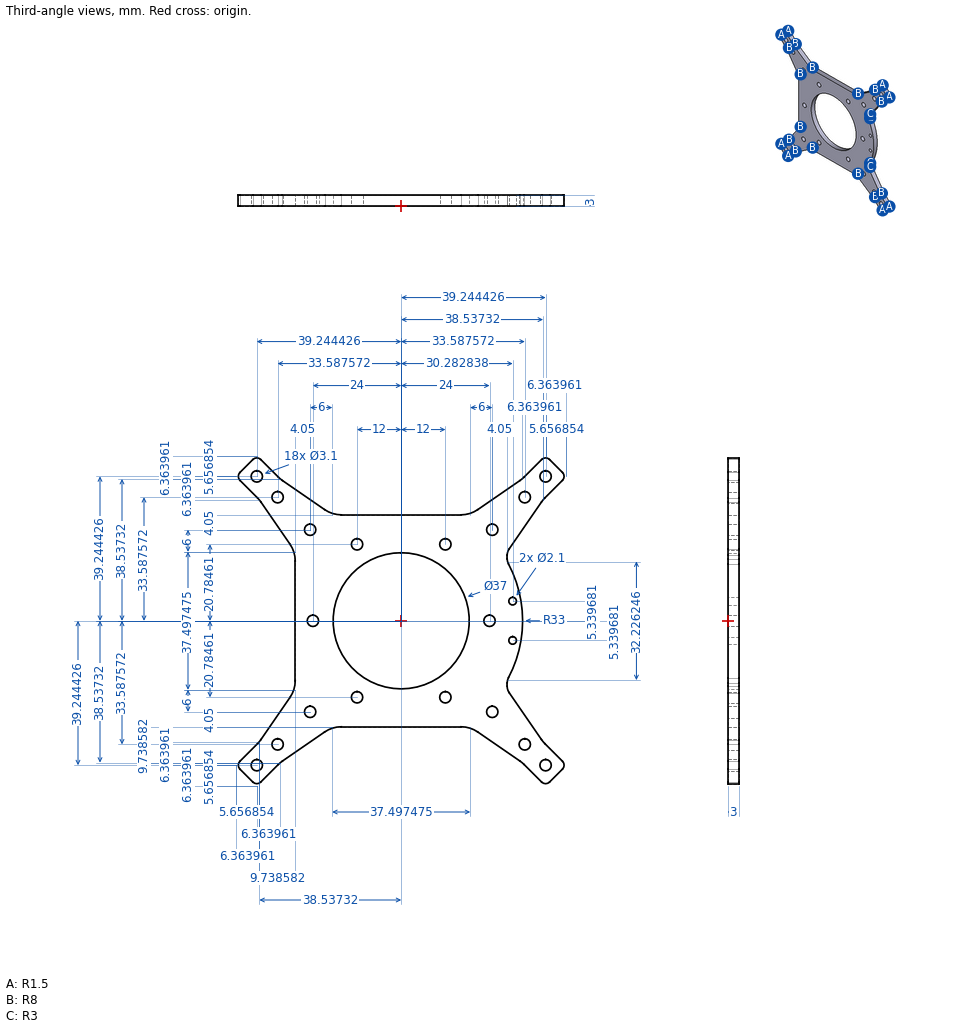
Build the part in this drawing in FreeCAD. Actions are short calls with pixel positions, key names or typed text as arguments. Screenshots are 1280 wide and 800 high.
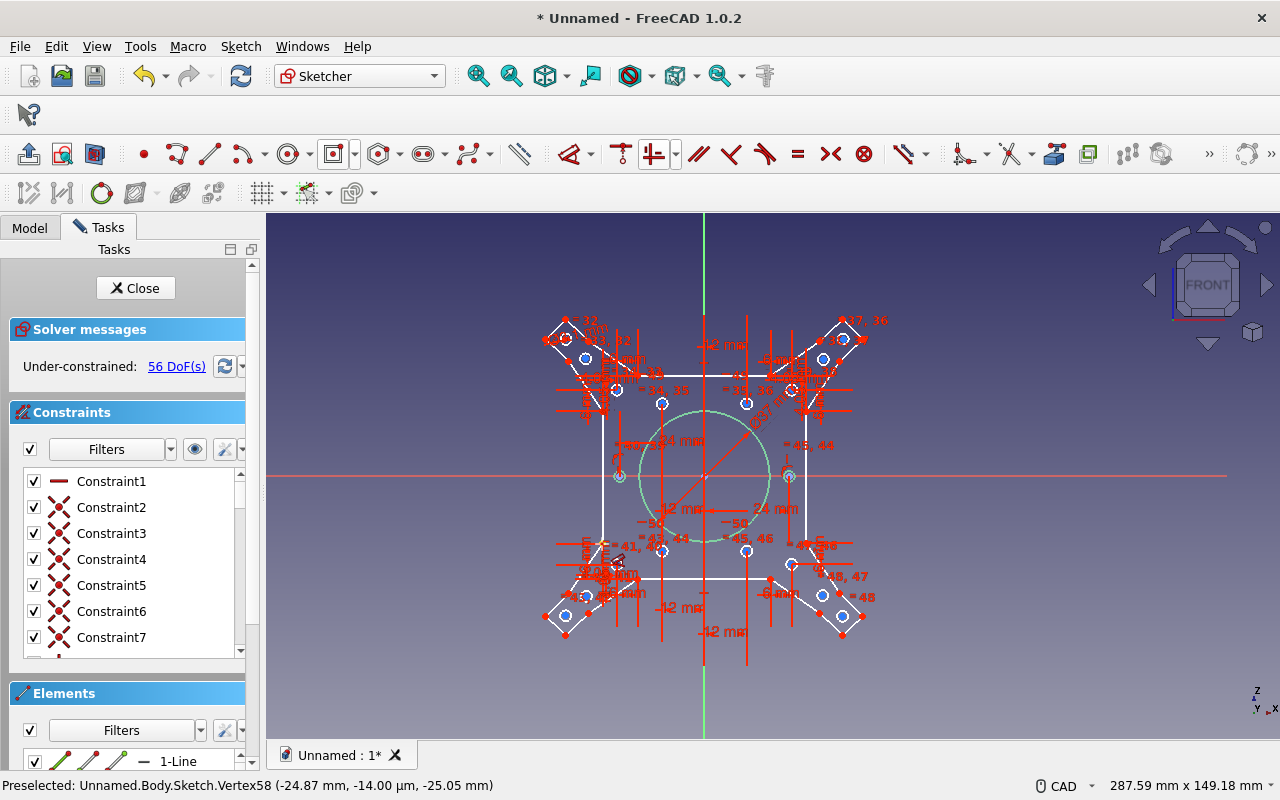
scroll(806, 543, up, 6)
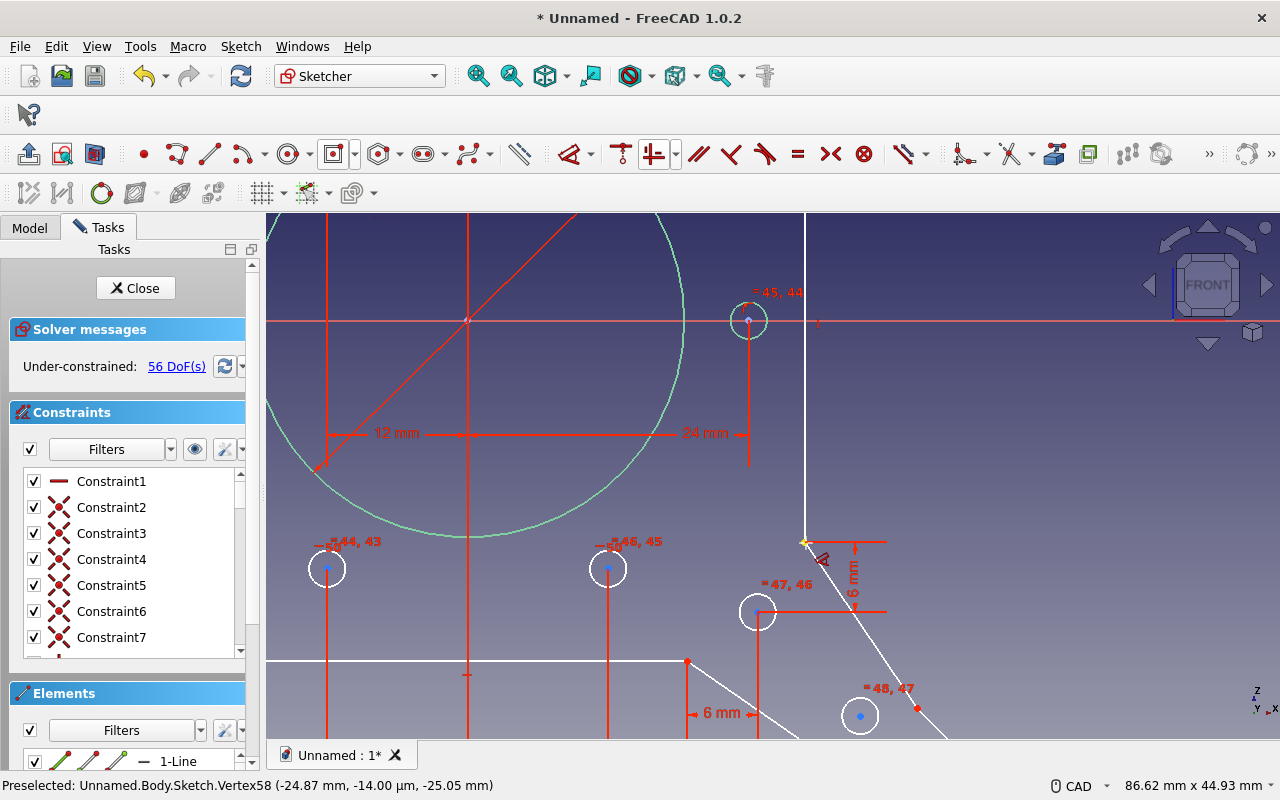
click(805, 542)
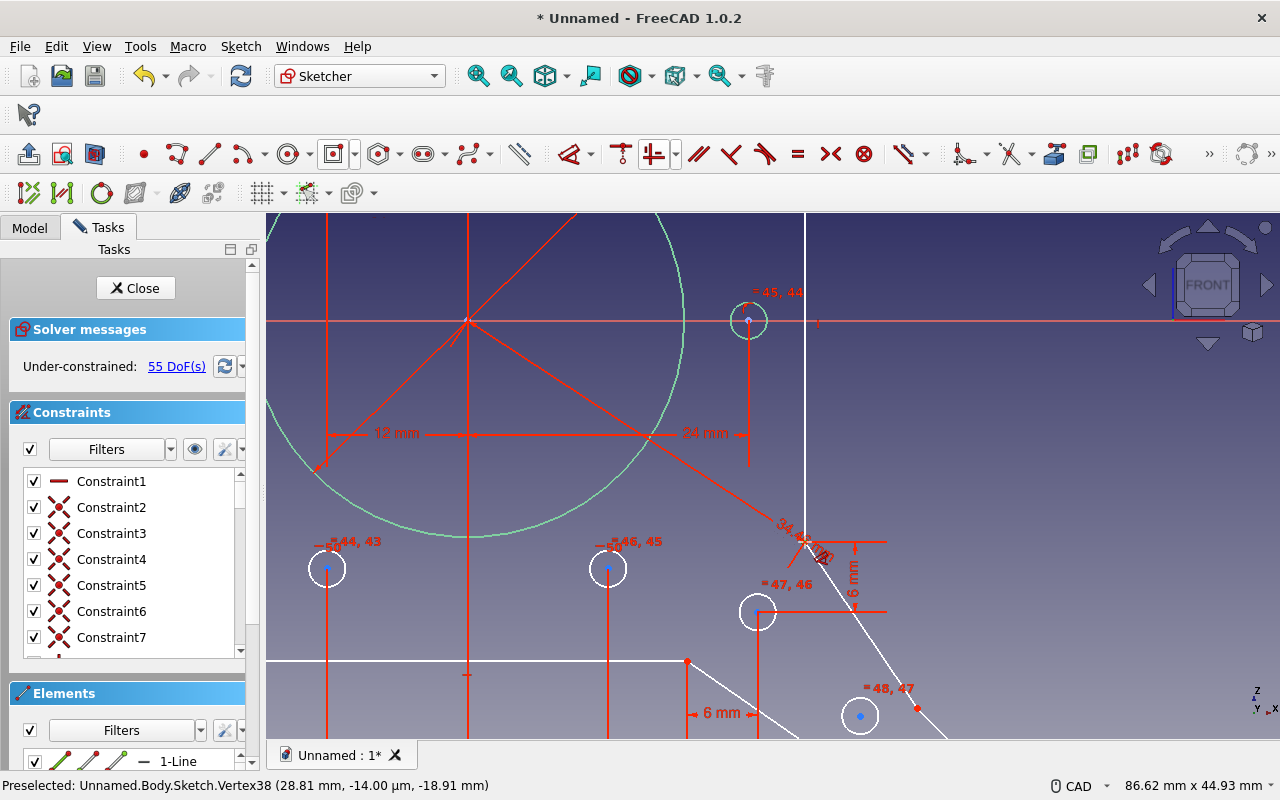
click(758, 612)
click(781, 646)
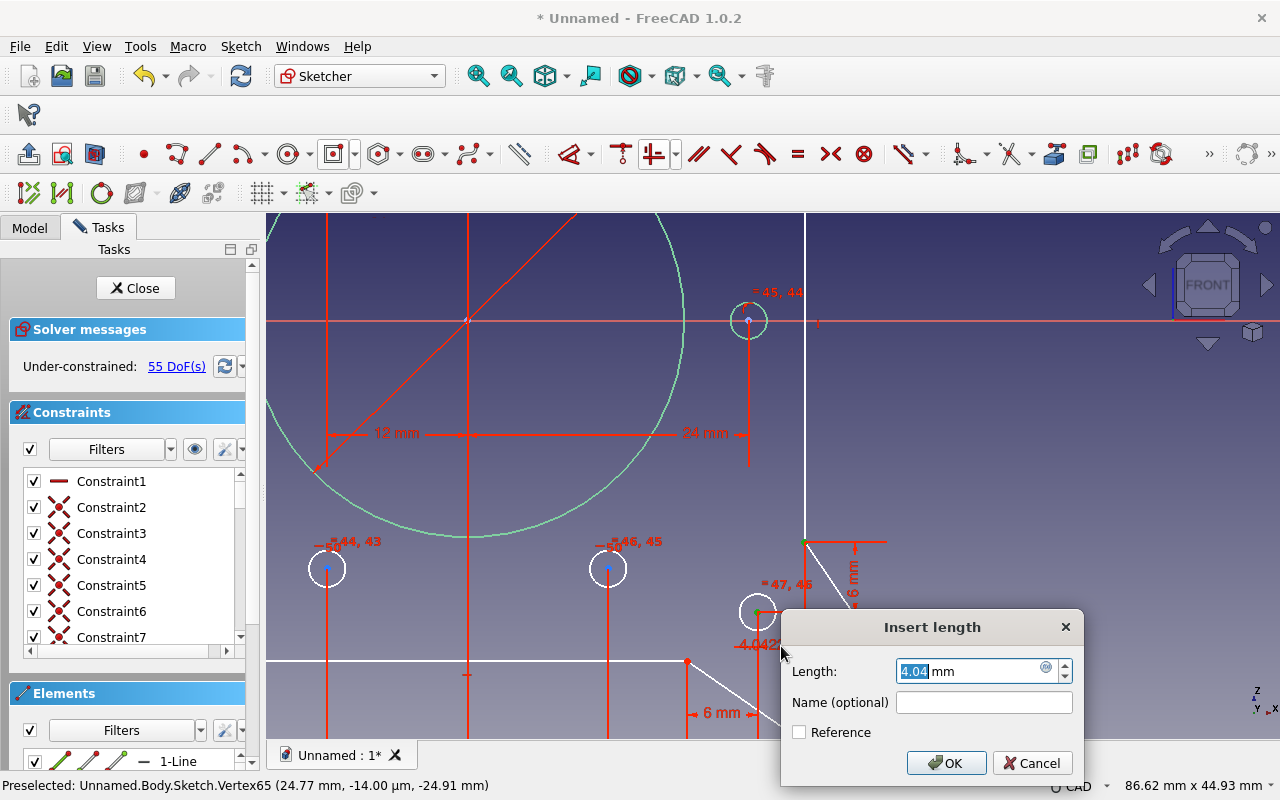
text(4.05)
key(Return)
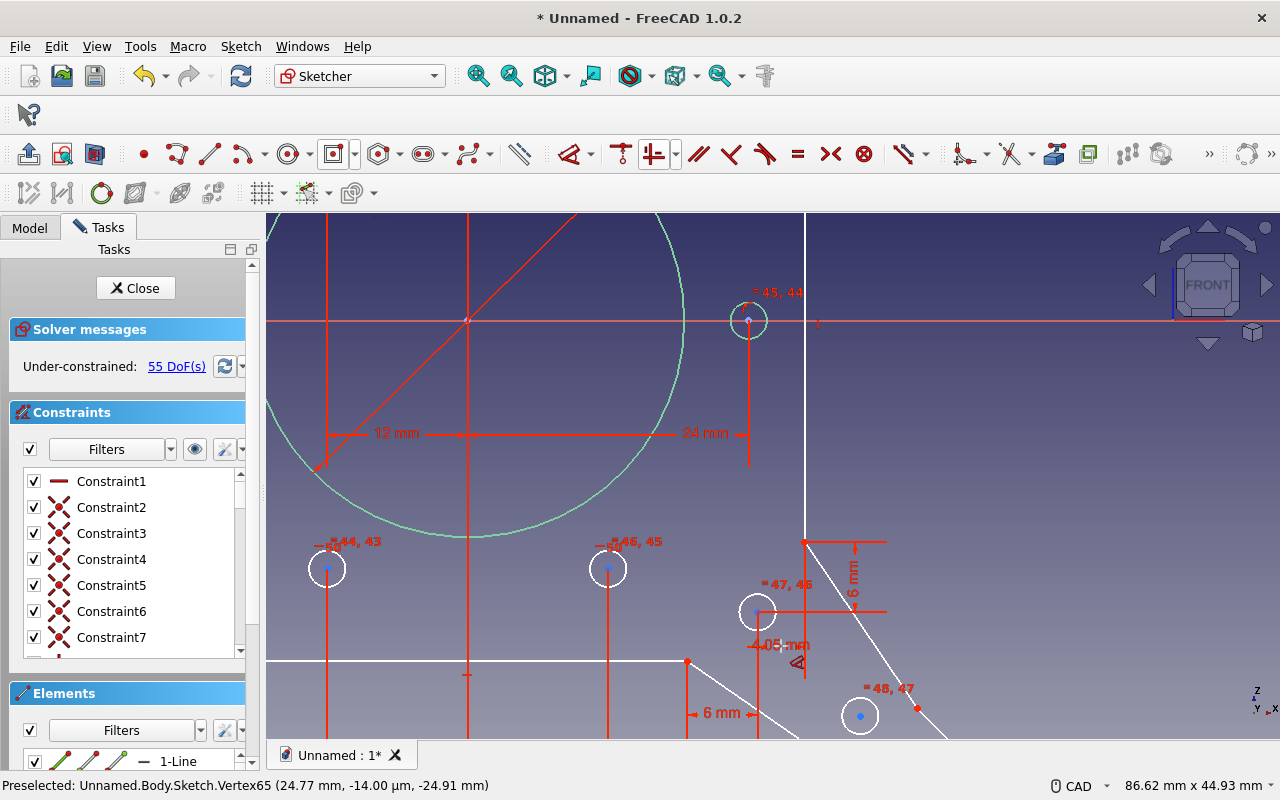
click(687, 661)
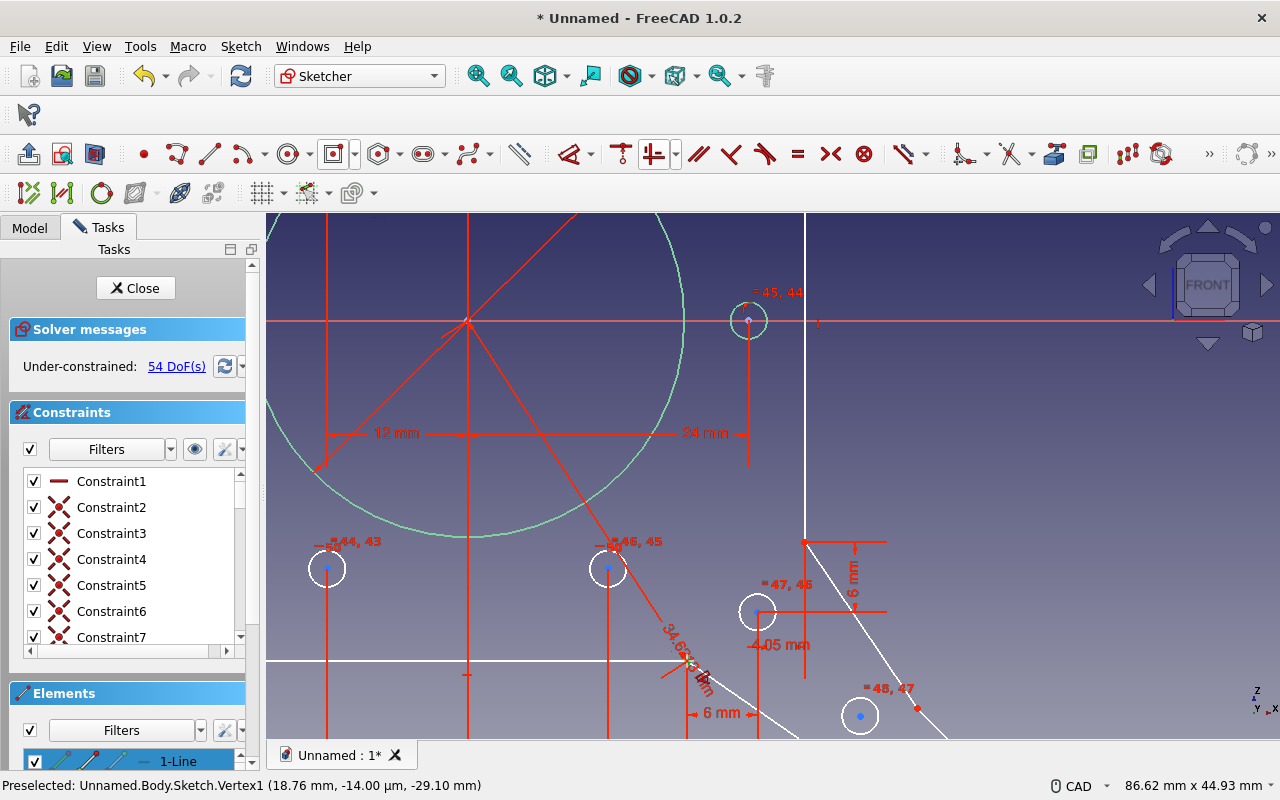
click(758, 612)
click(792, 626)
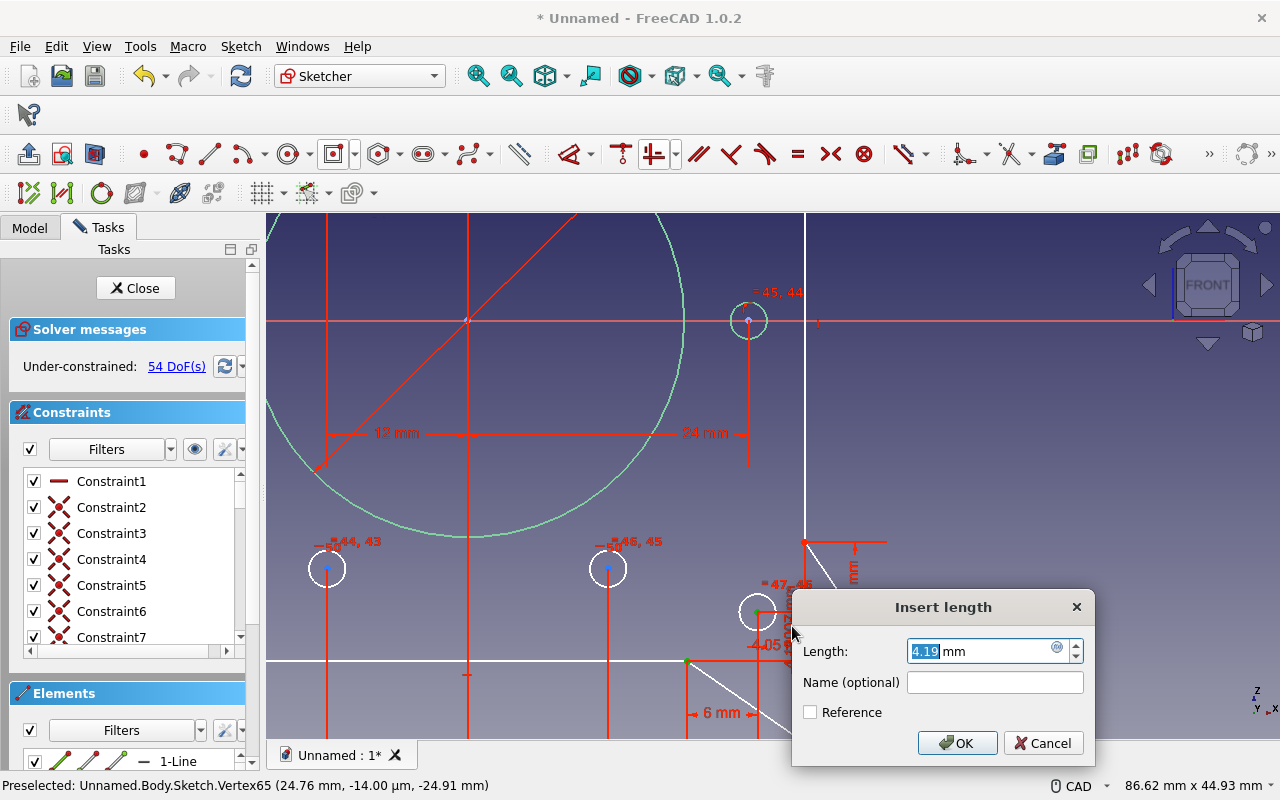
text(4.05)
key(Return)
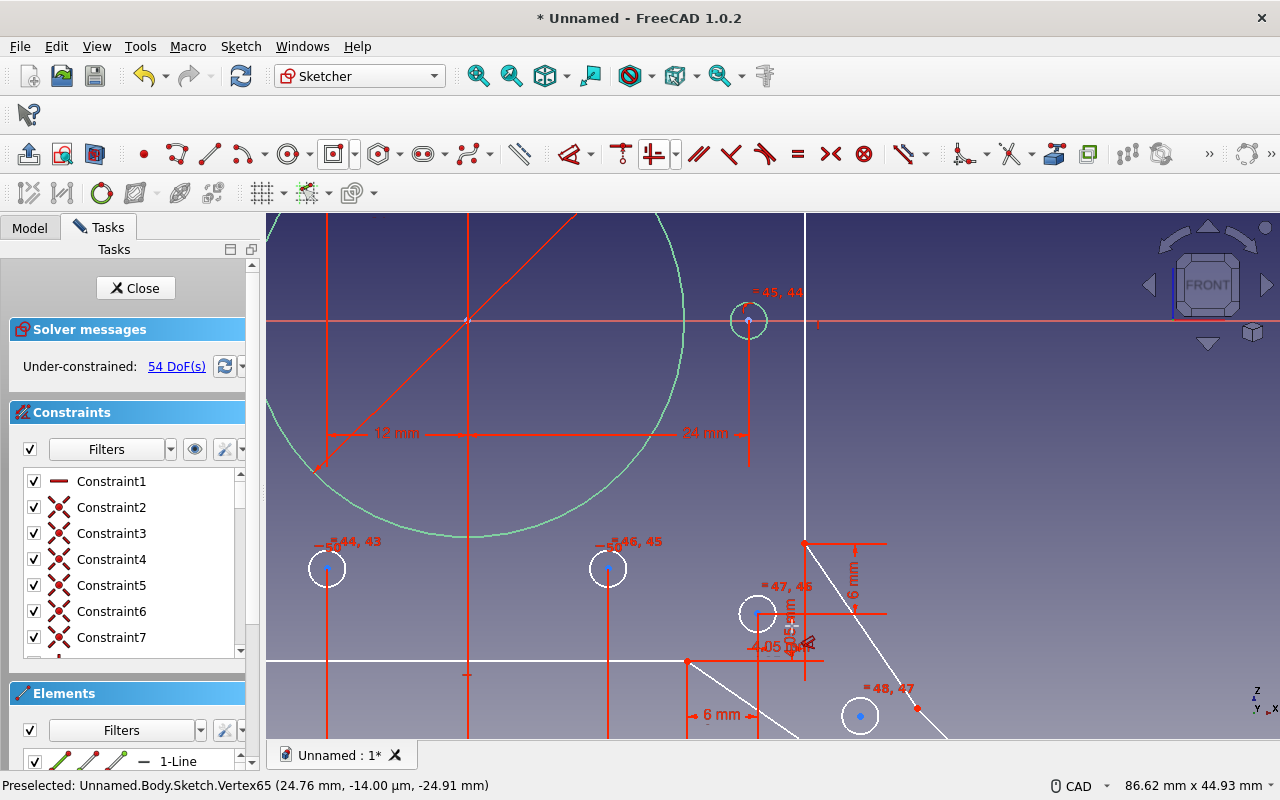
scroll(807, 543, down, 6)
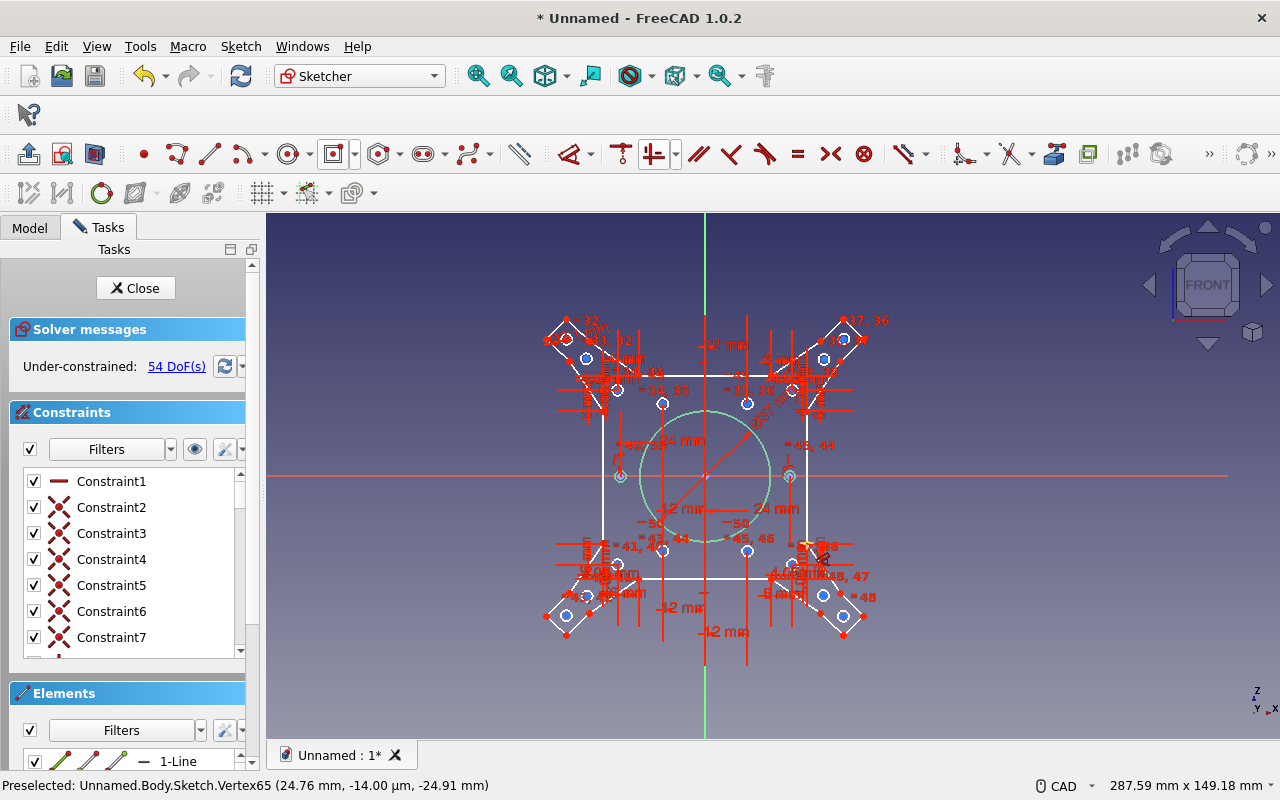
click(663, 404)
click(581, 440)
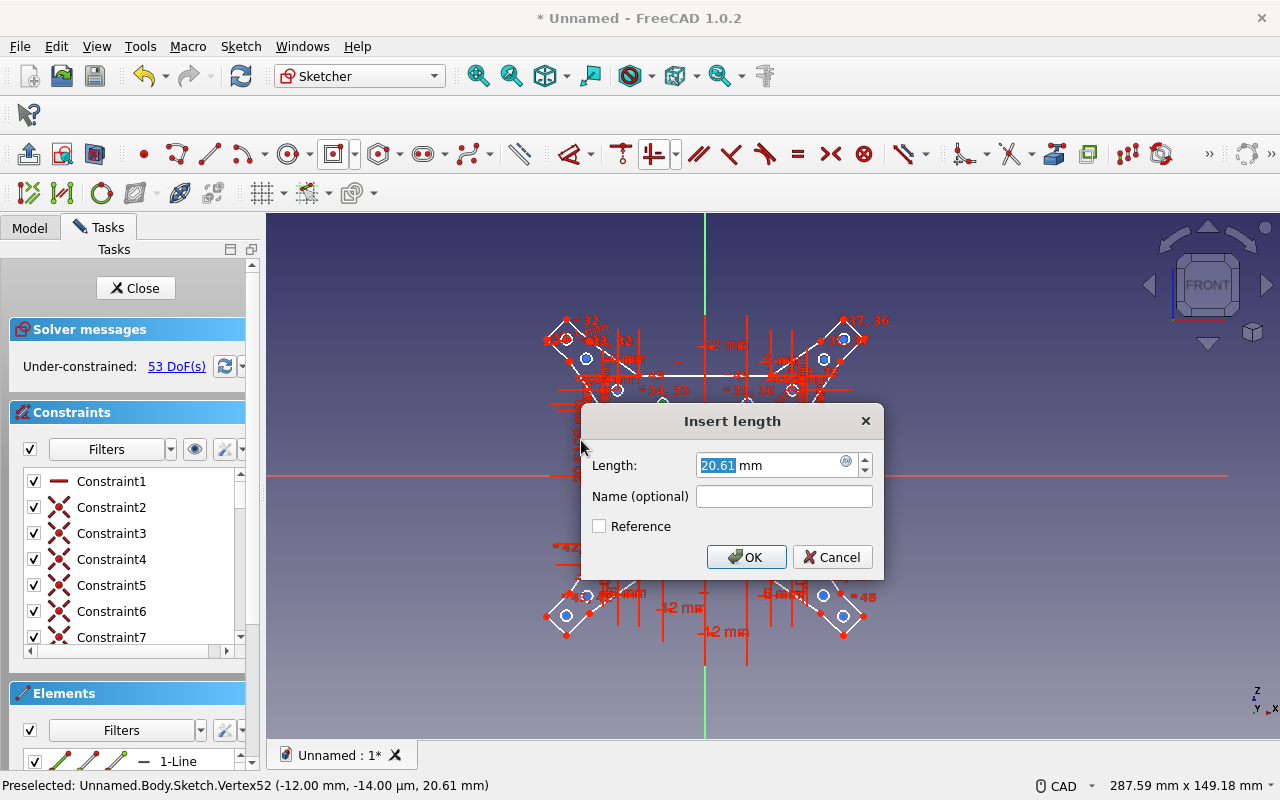
text(20.78461)
key(Return)